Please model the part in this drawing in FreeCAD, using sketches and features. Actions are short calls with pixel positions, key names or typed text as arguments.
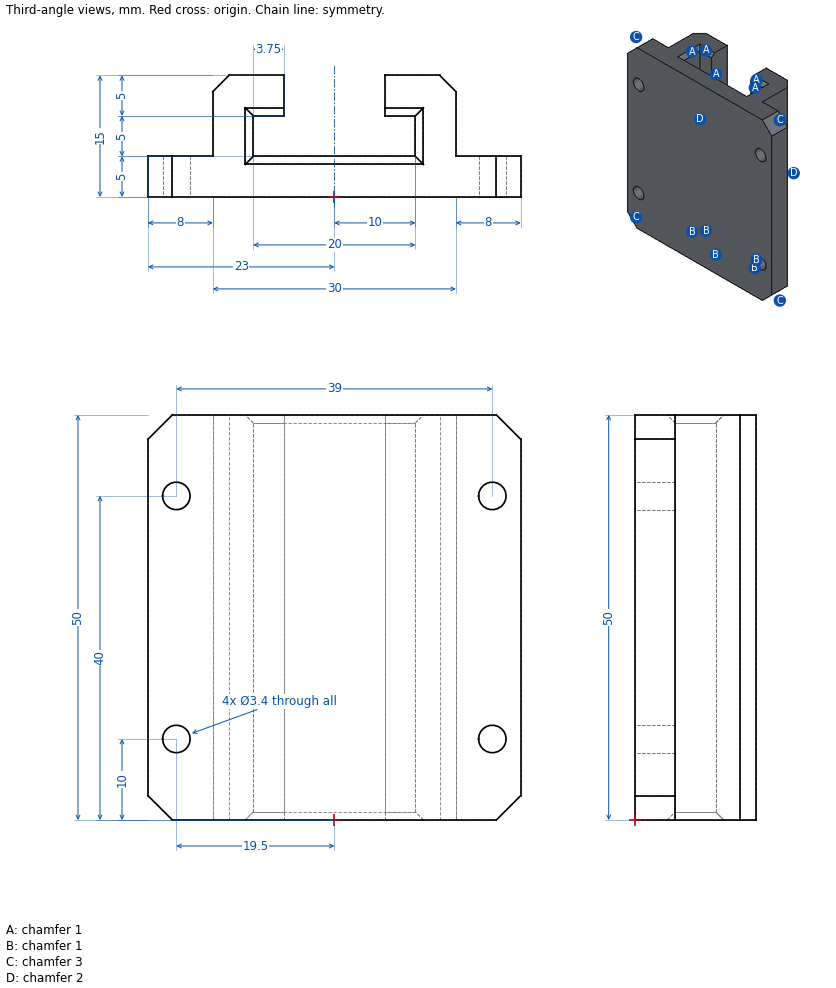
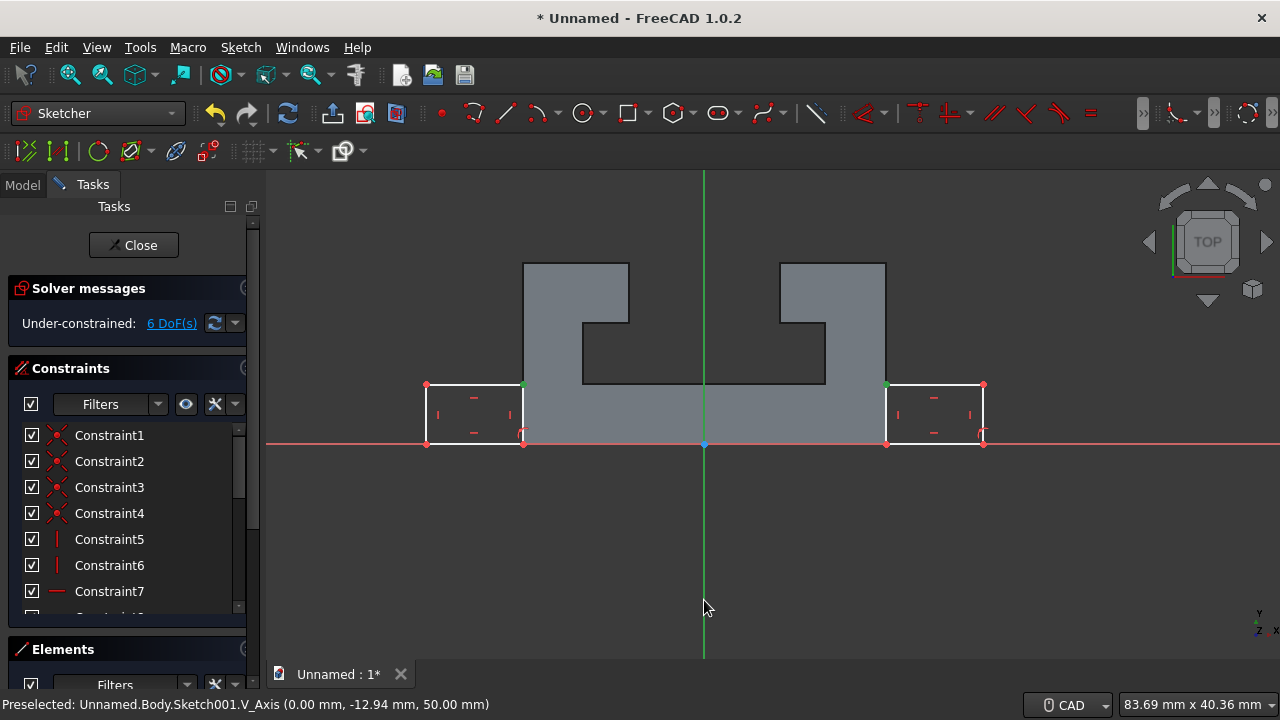
key(s)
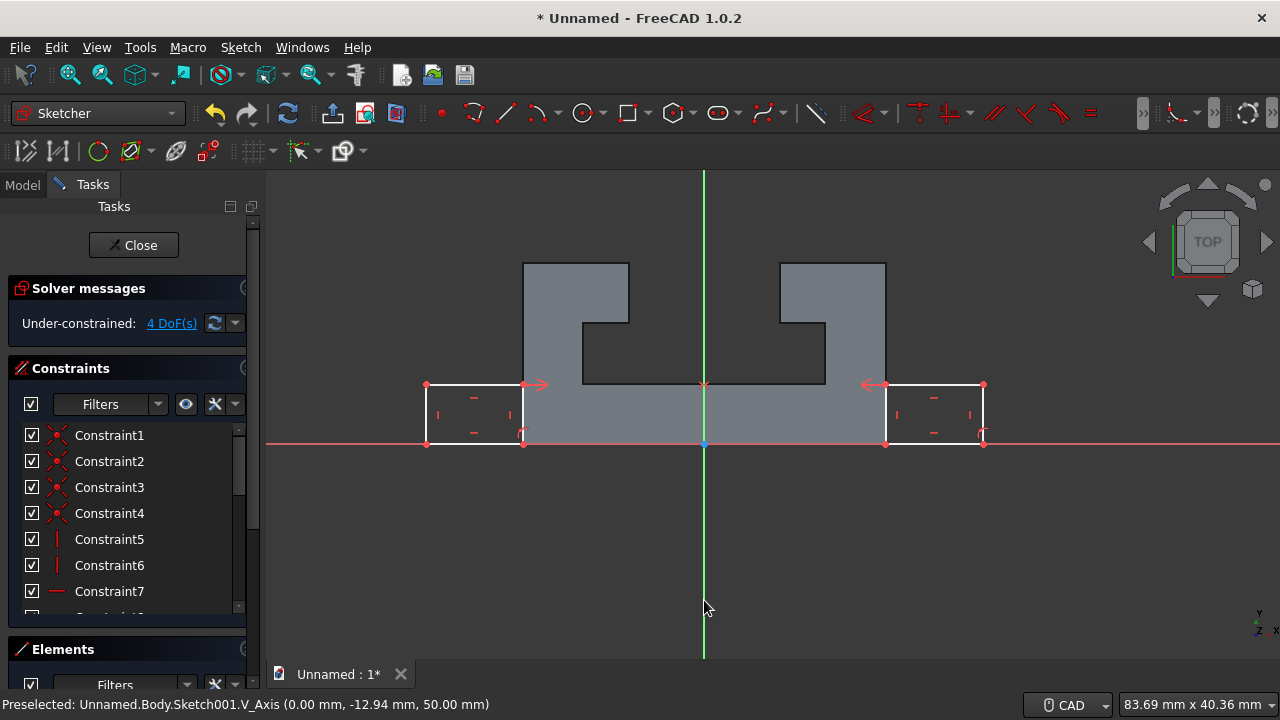
key(d)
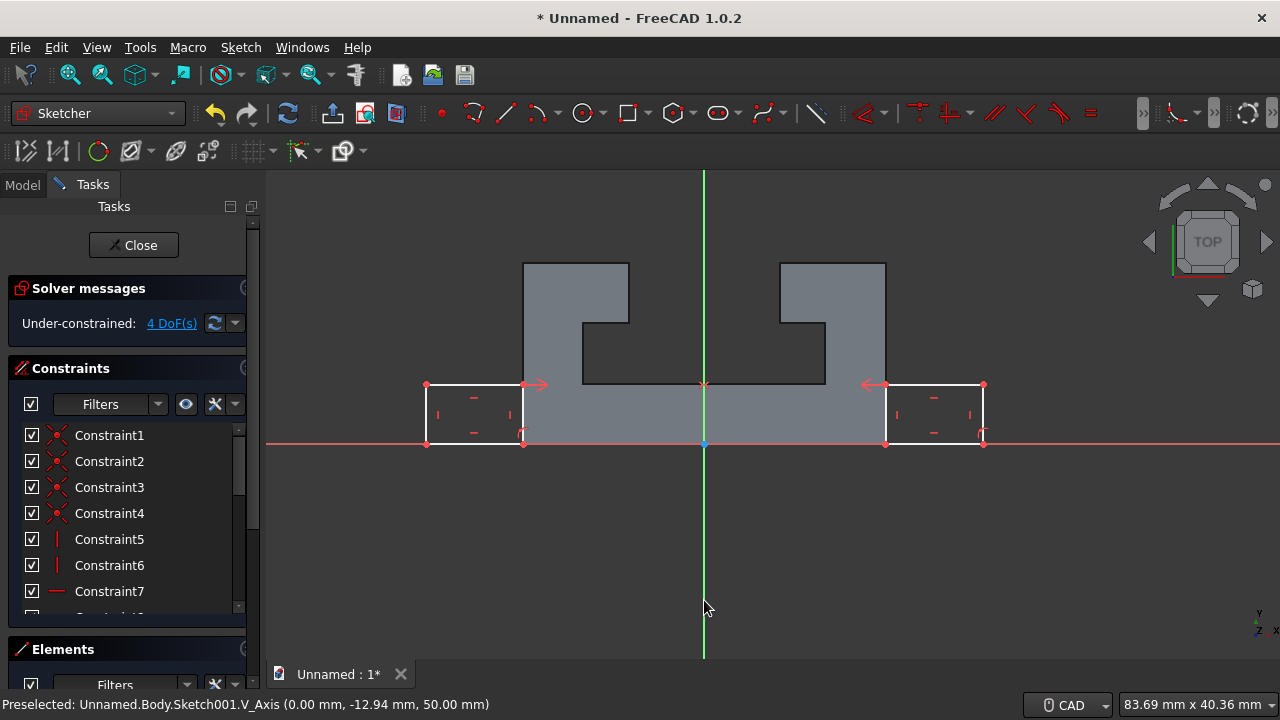
click(426, 403)
click(392, 415)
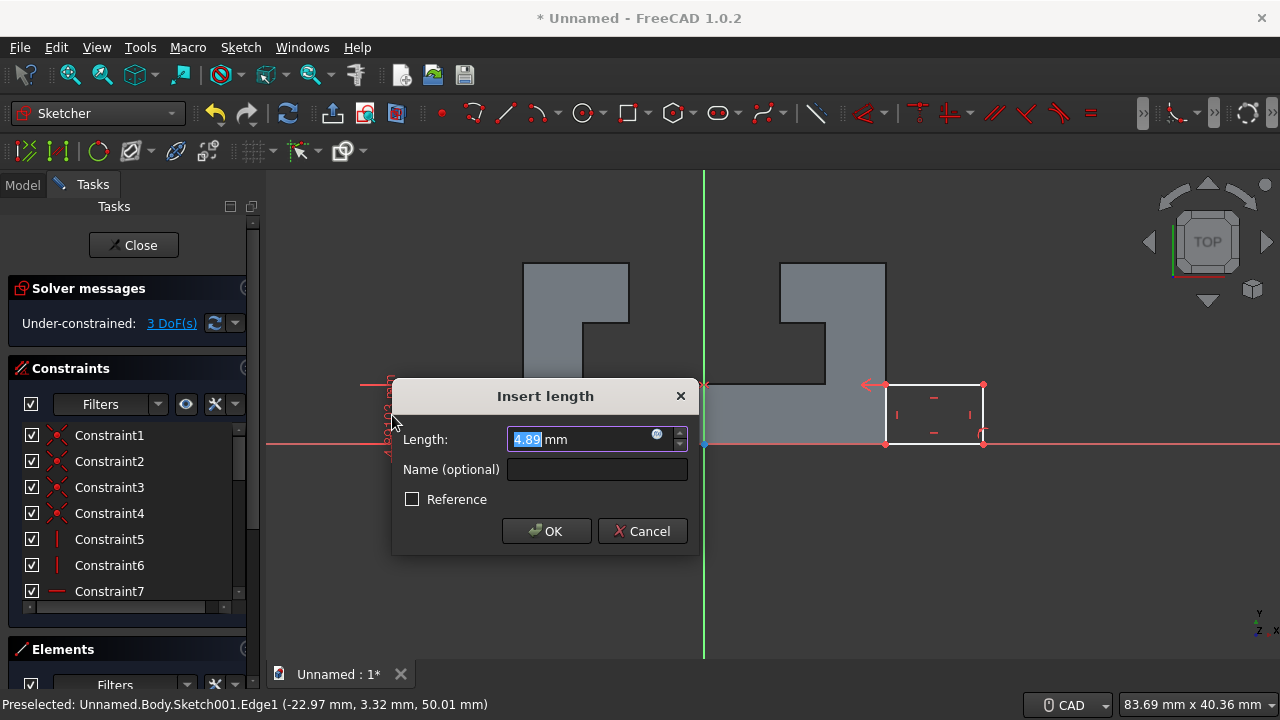
text(5)
key(Return)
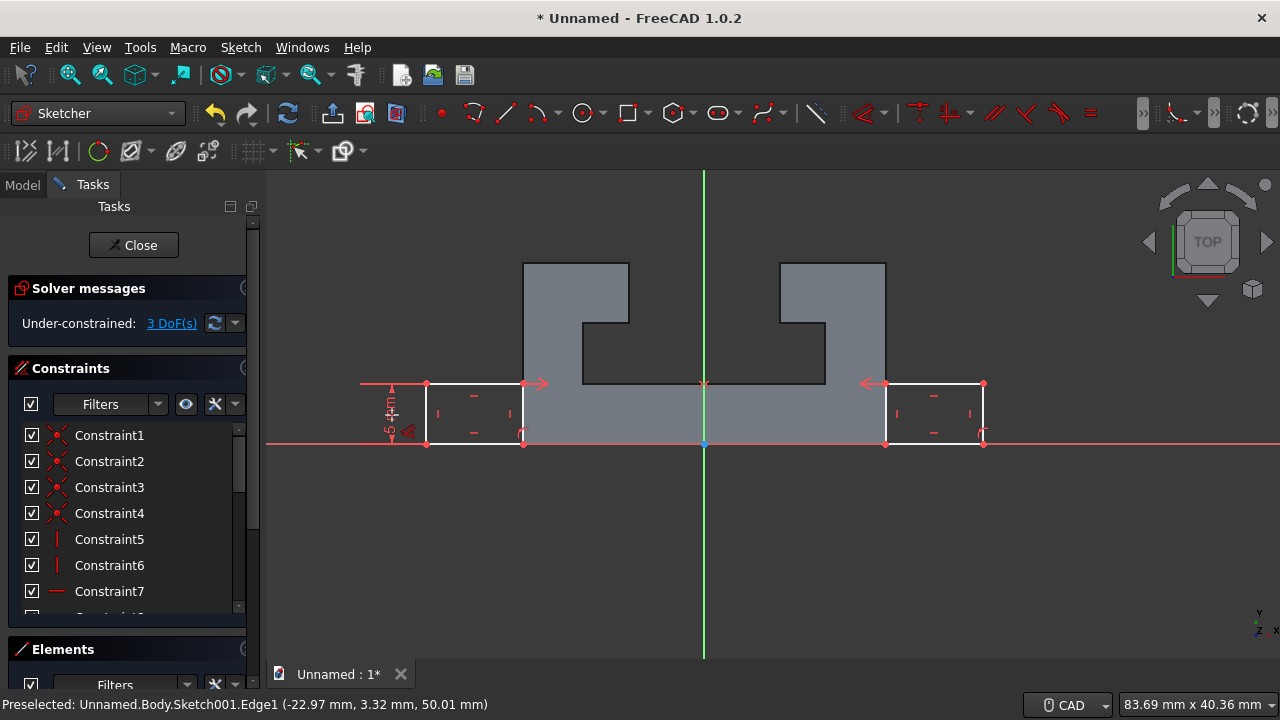
click(455, 444)
click(475, 478)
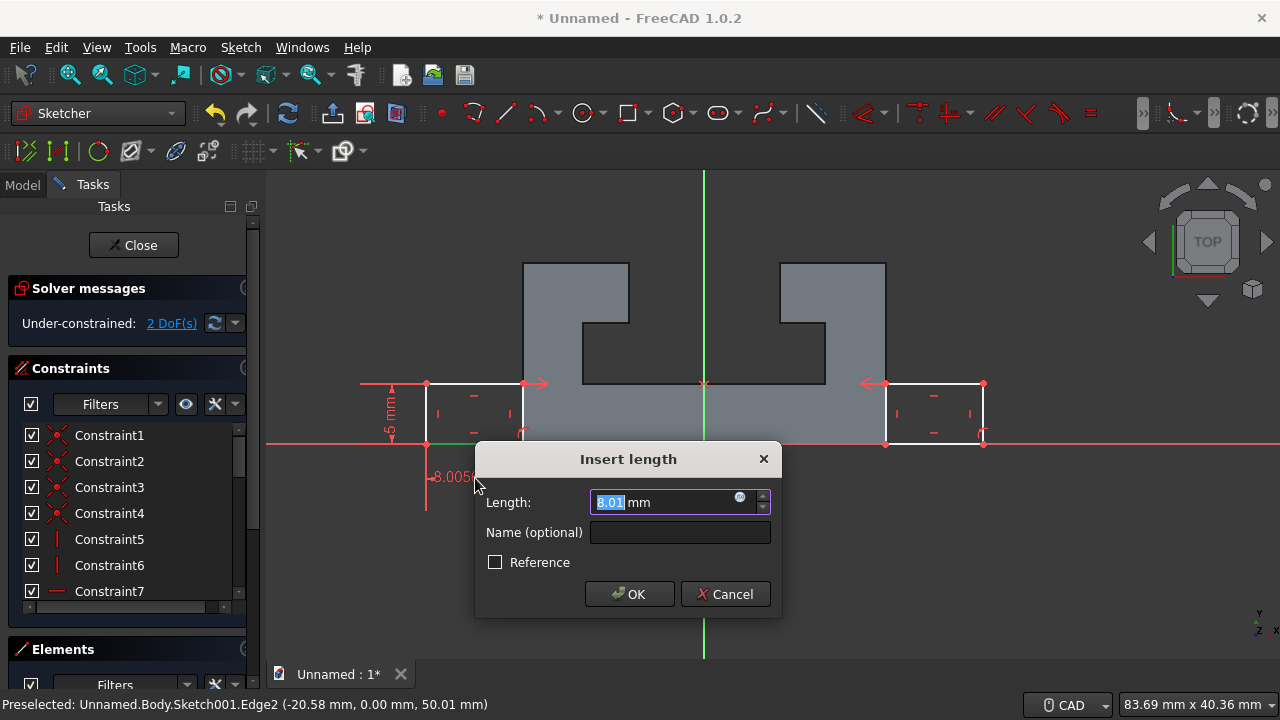
text(8)
key(Return)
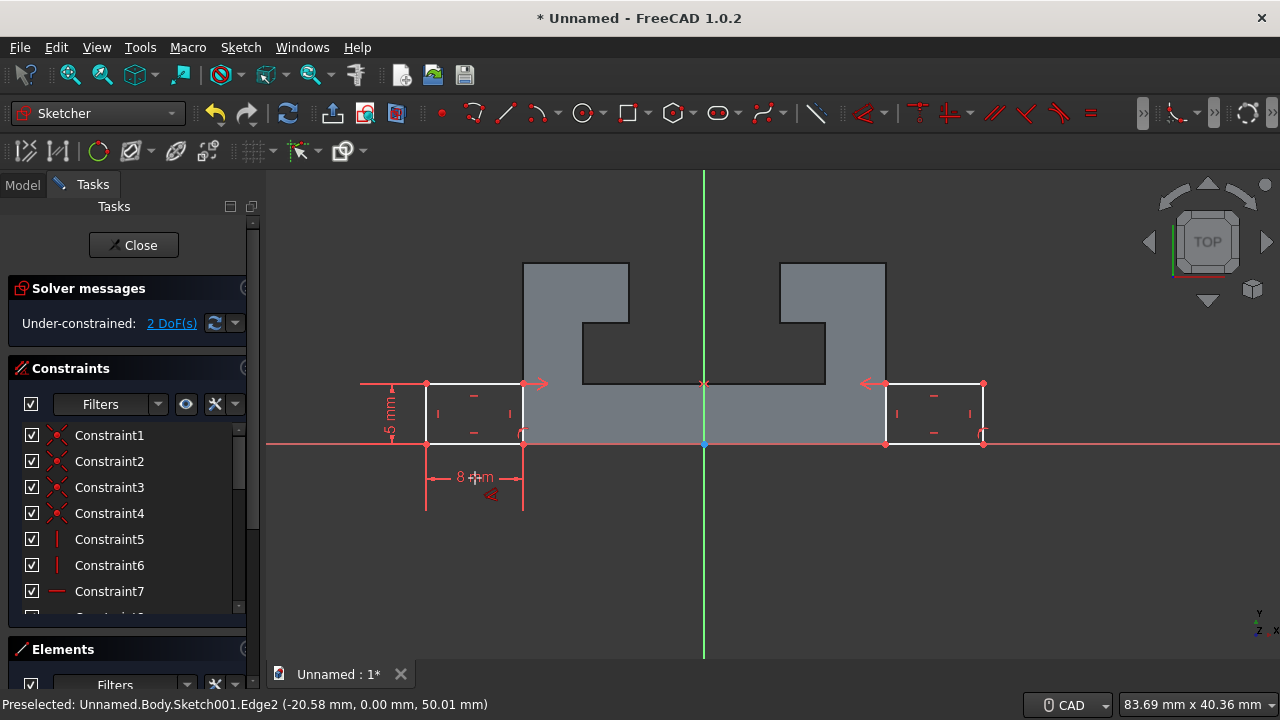
click(915, 444)
click(934, 478)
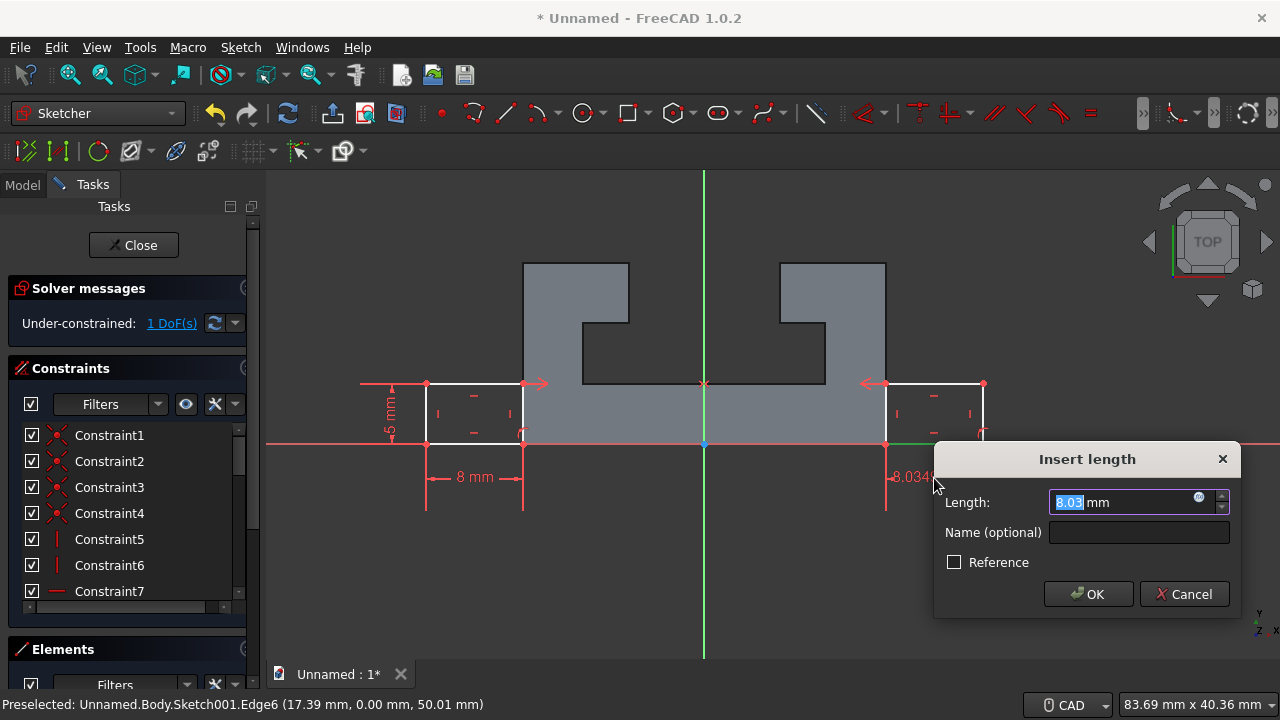
text(8)
key(Return)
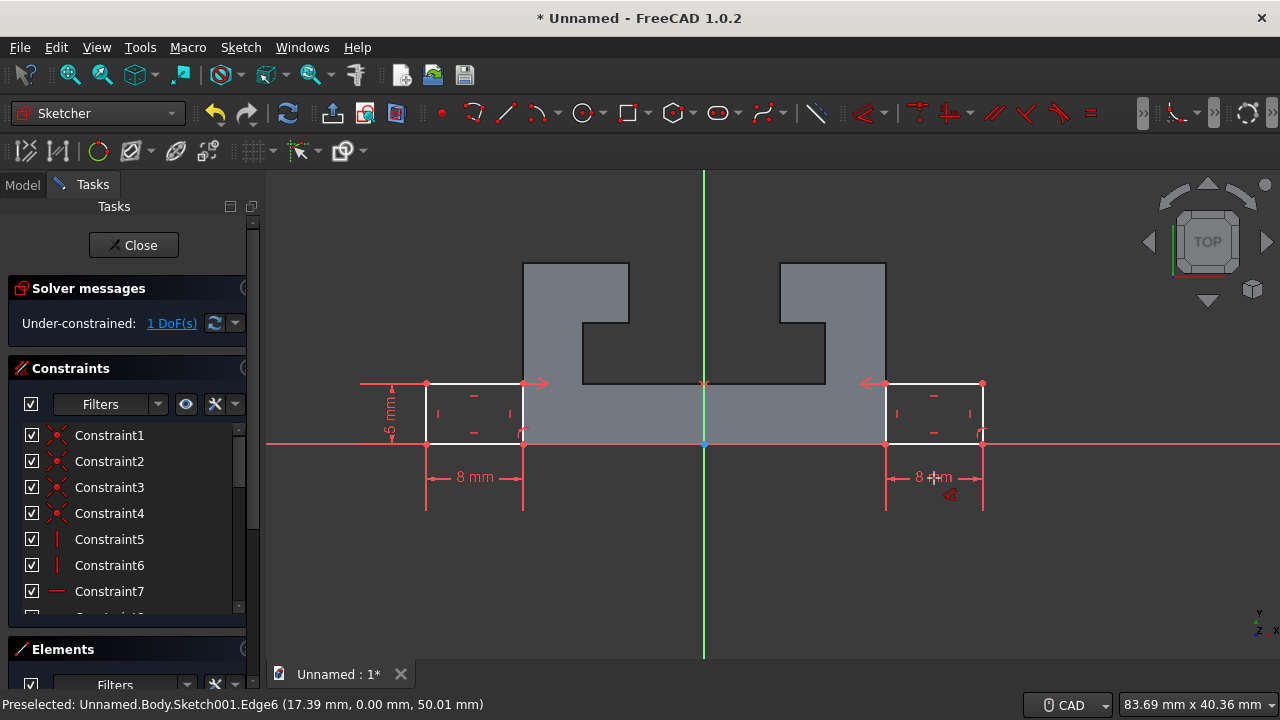
click(426, 384)
click(565, 350)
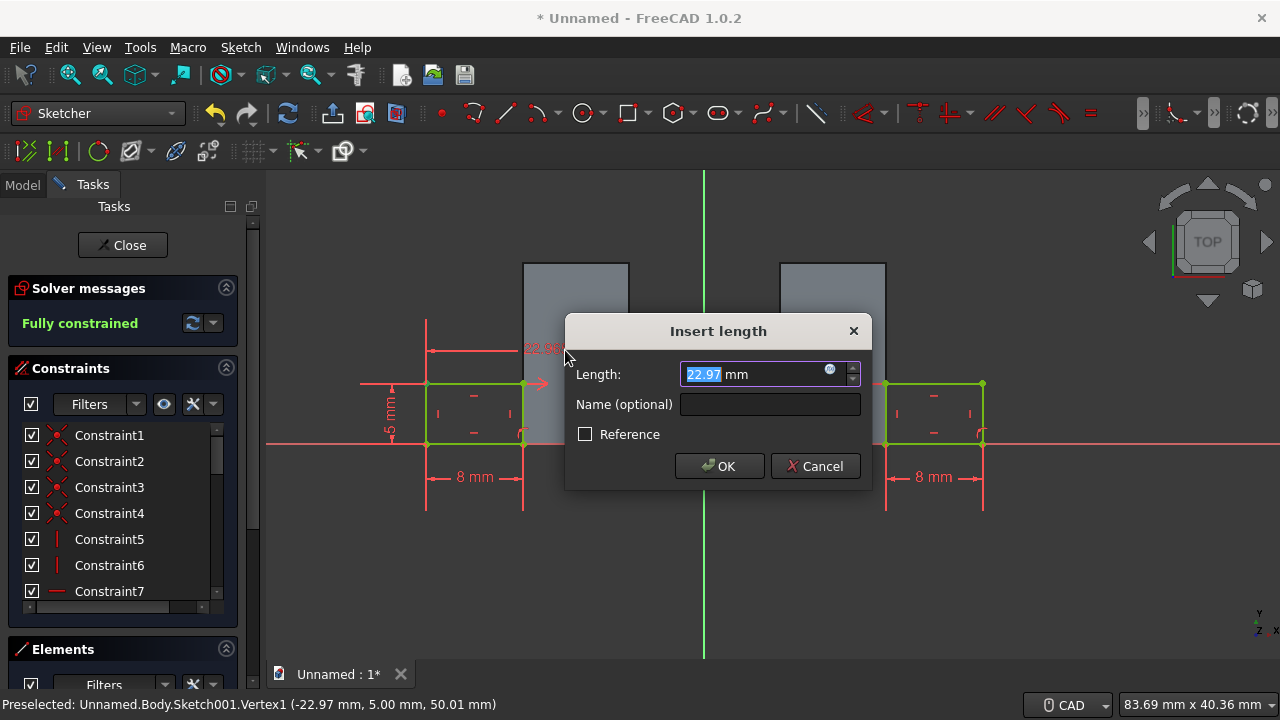
text(23)
key(Return)
key(Escape)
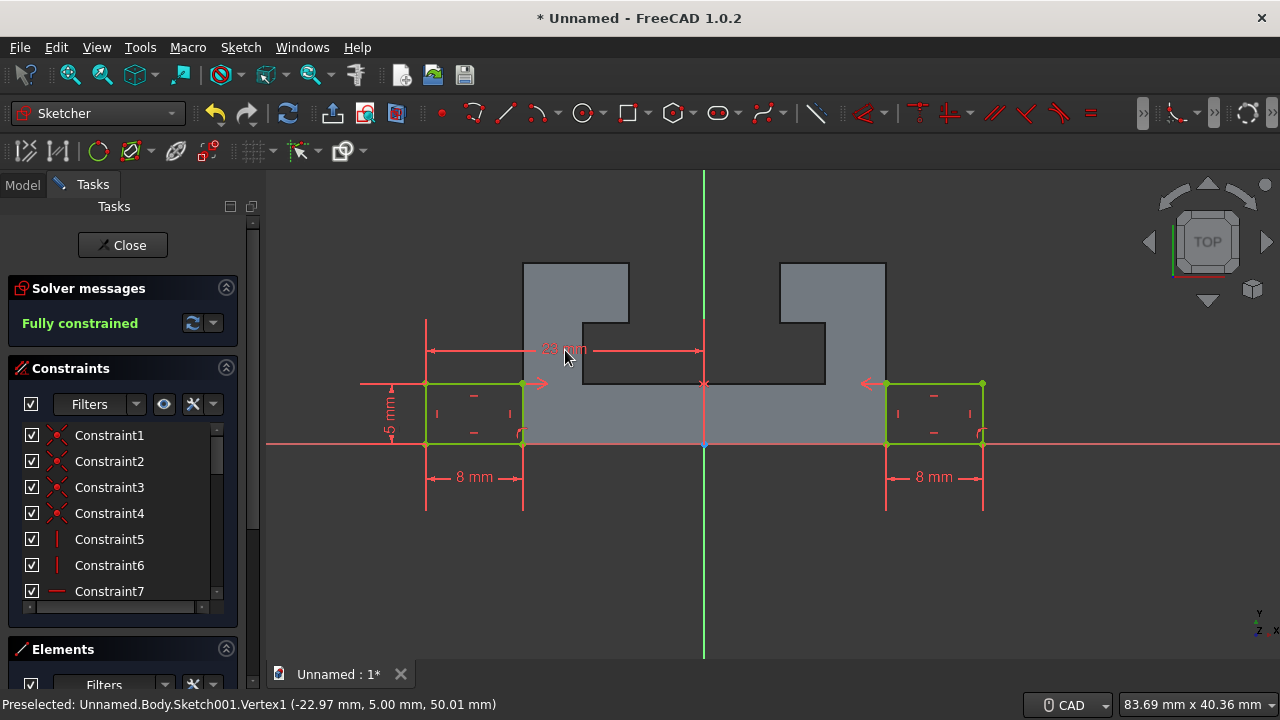
click(123, 245)